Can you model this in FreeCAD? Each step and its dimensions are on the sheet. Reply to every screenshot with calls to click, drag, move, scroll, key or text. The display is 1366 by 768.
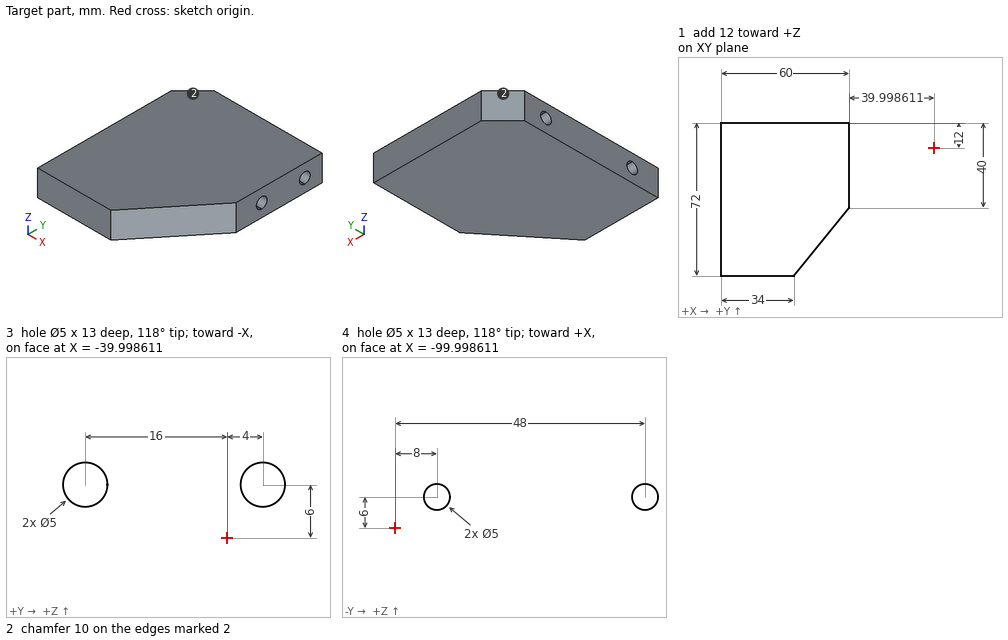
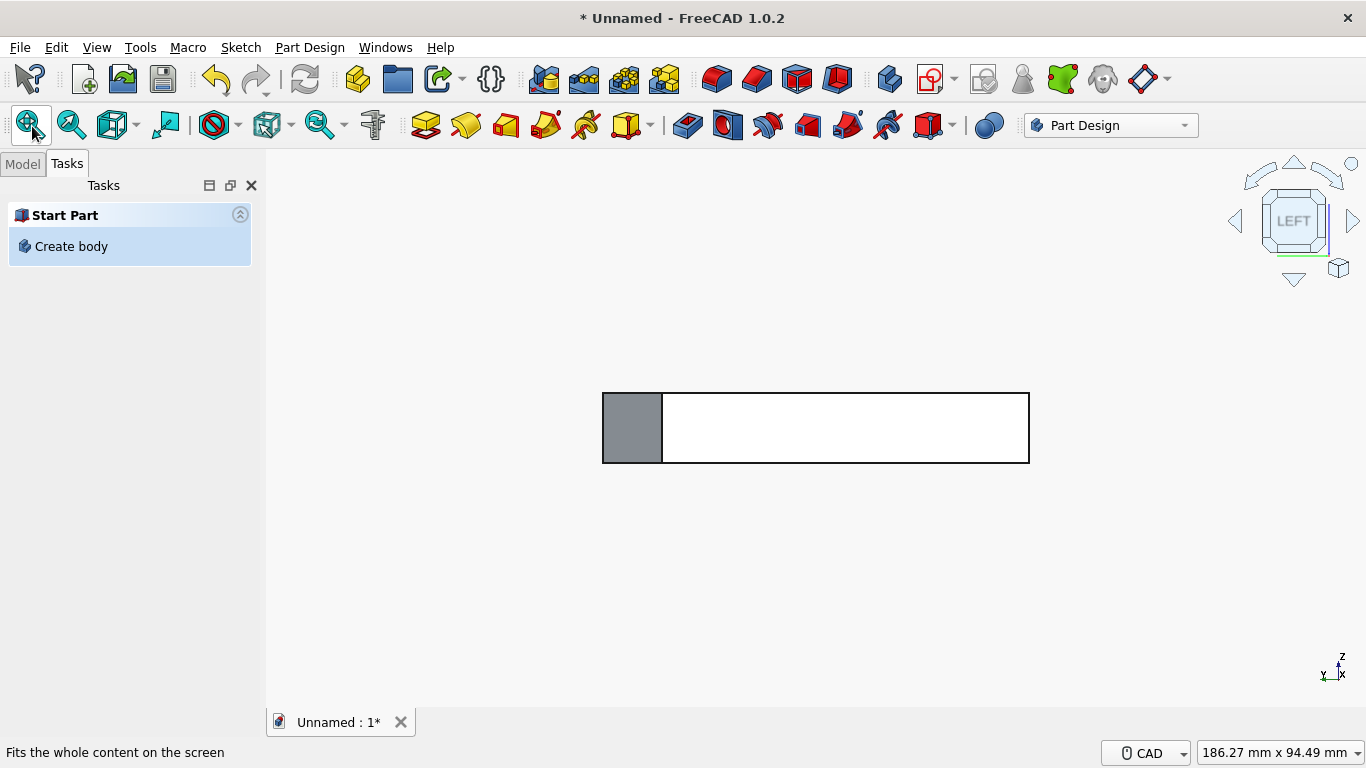
click(741, 427)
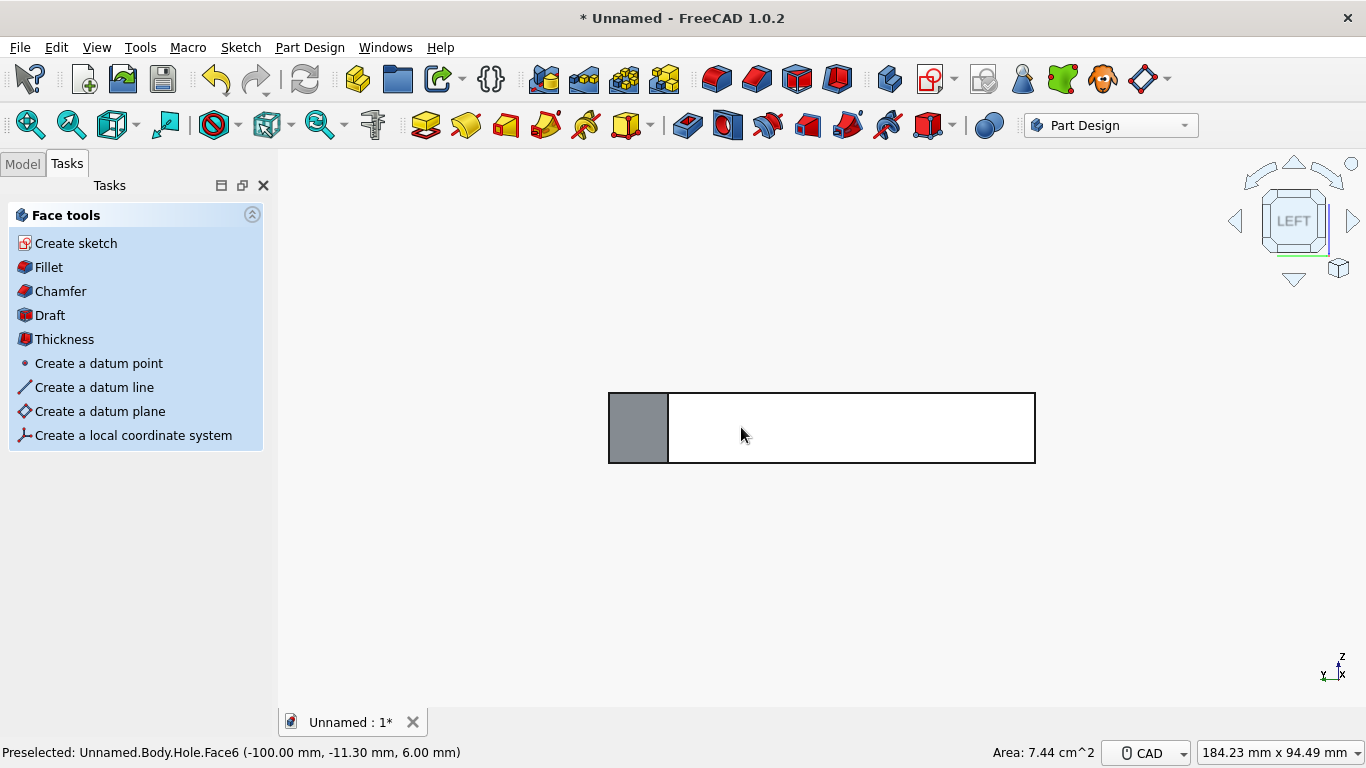
click(930, 80)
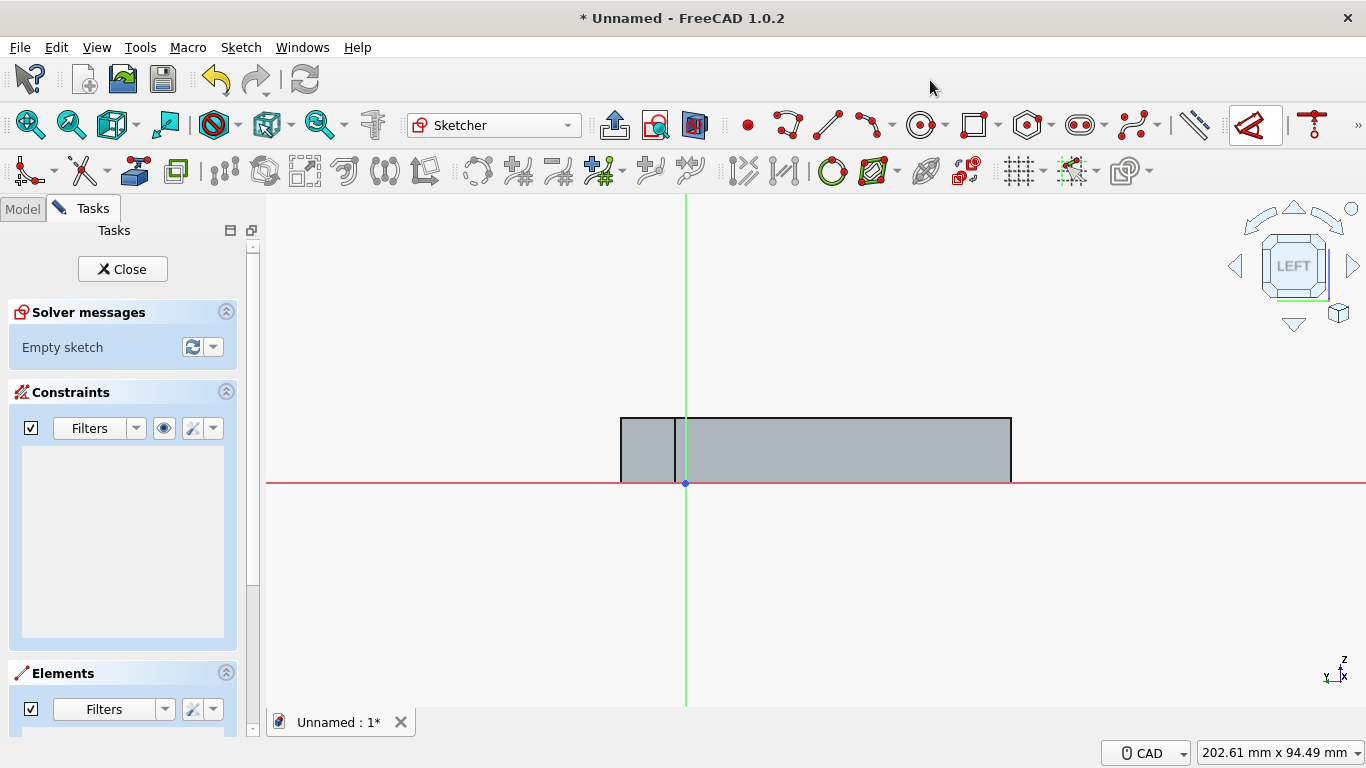
scroll(884, 468, up, 4)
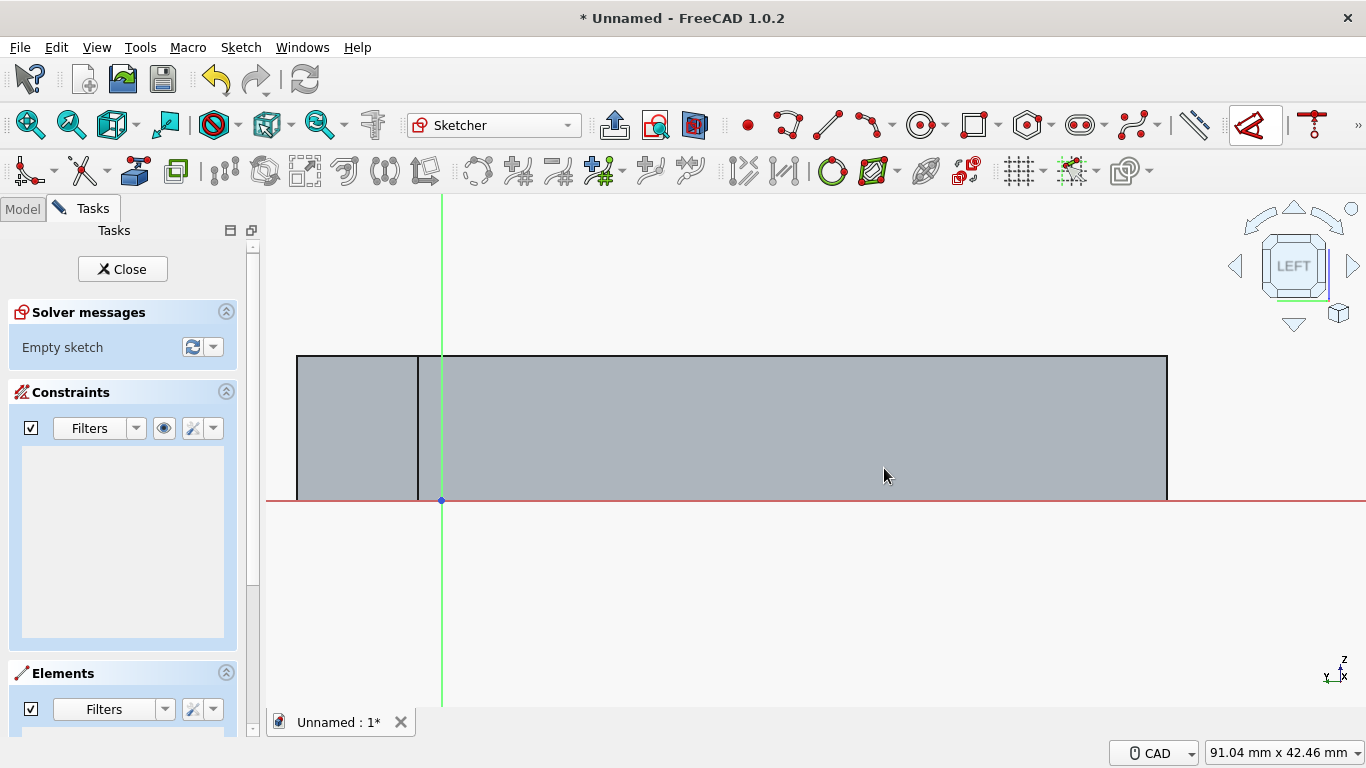
key(g)
key(c)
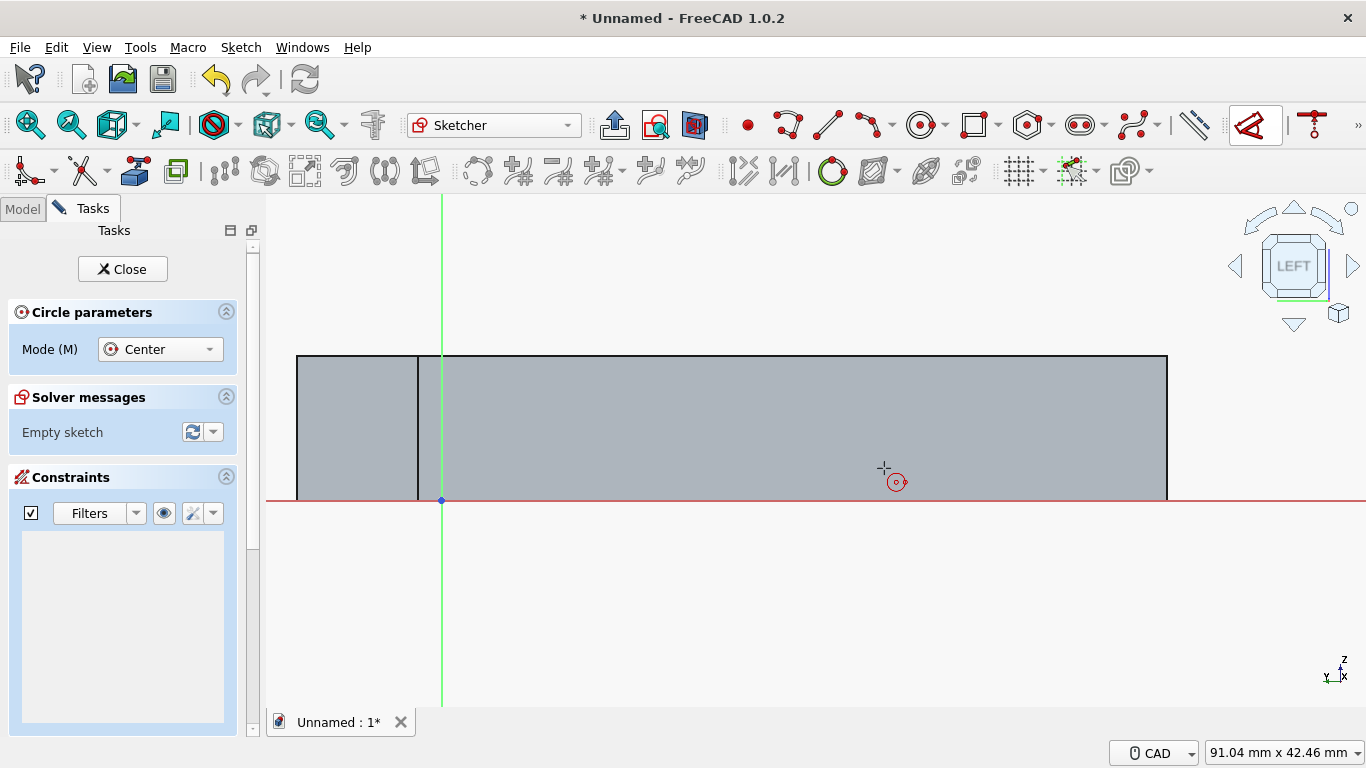
click(539, 428)
move(560, 407)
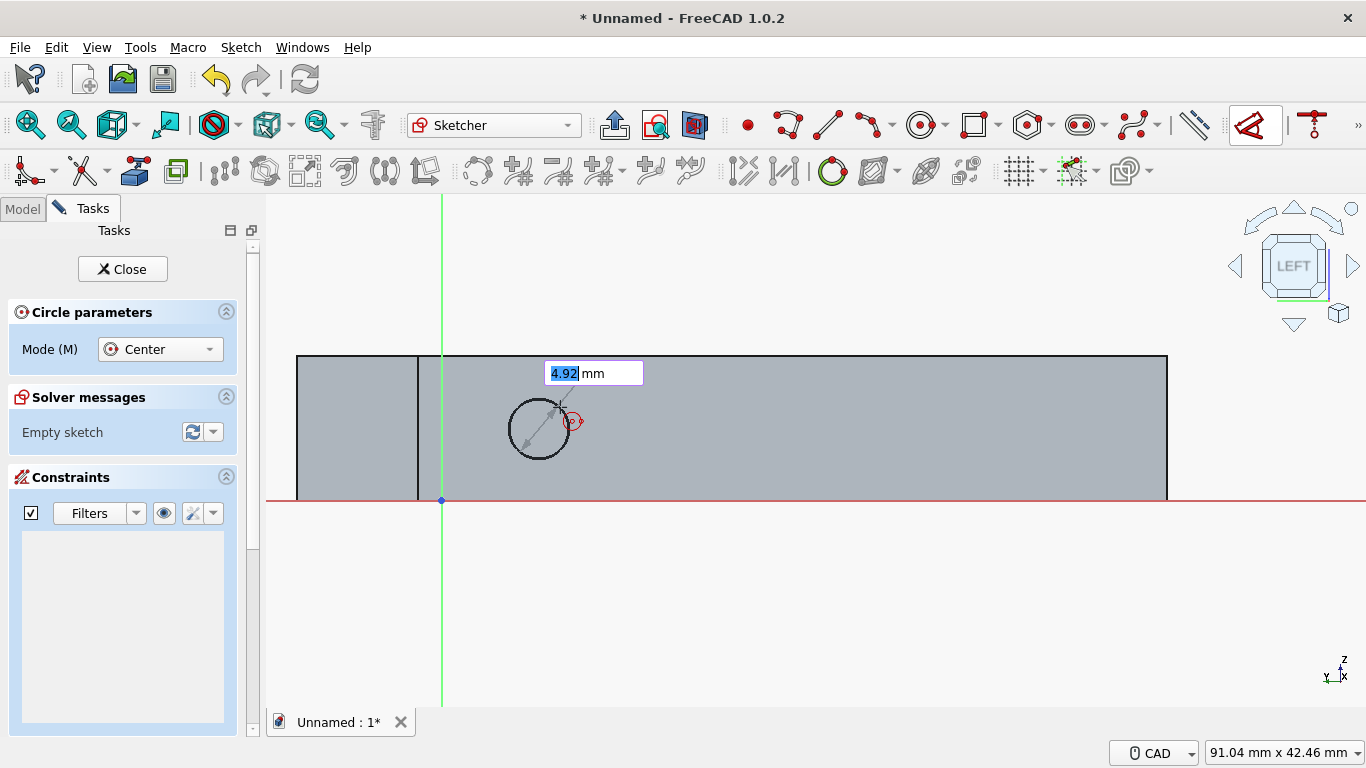
text(5)
key(Return)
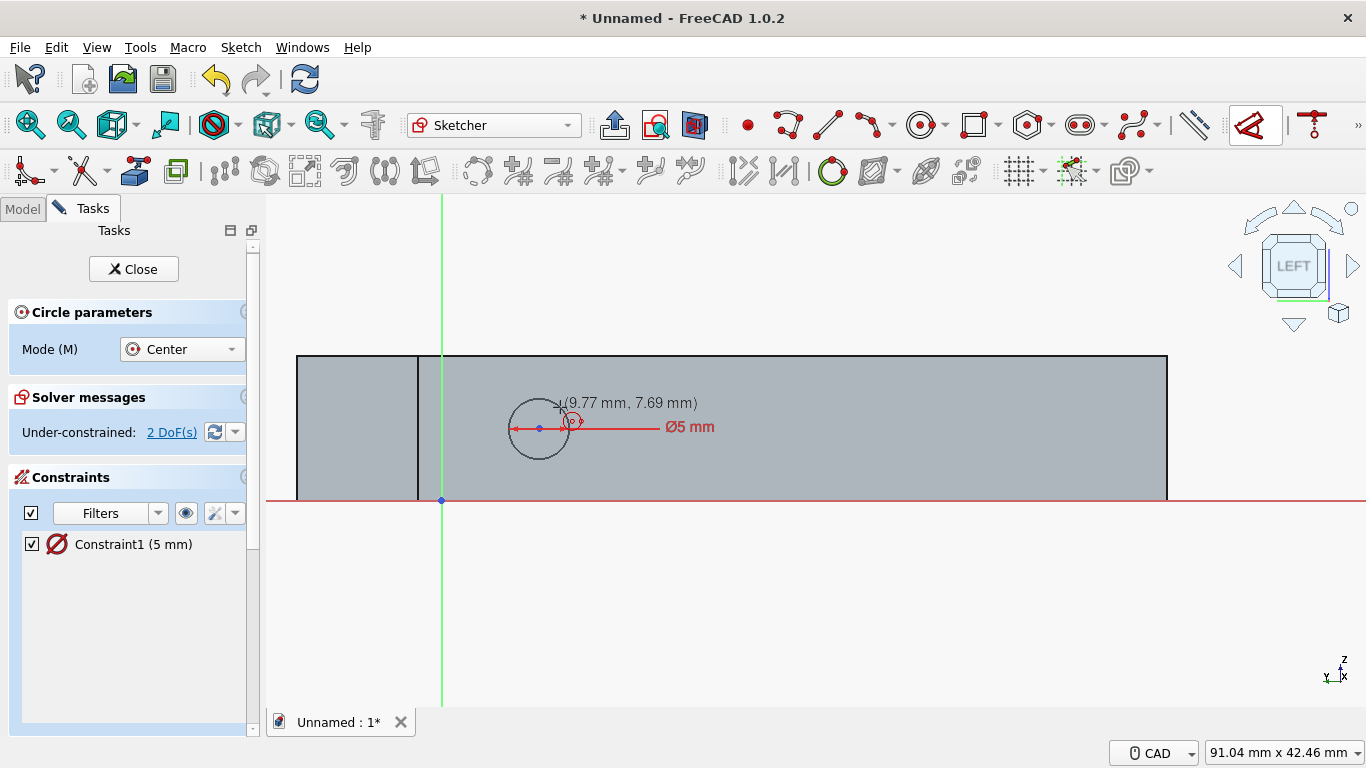
click(1022, 428)
move(1043, 407)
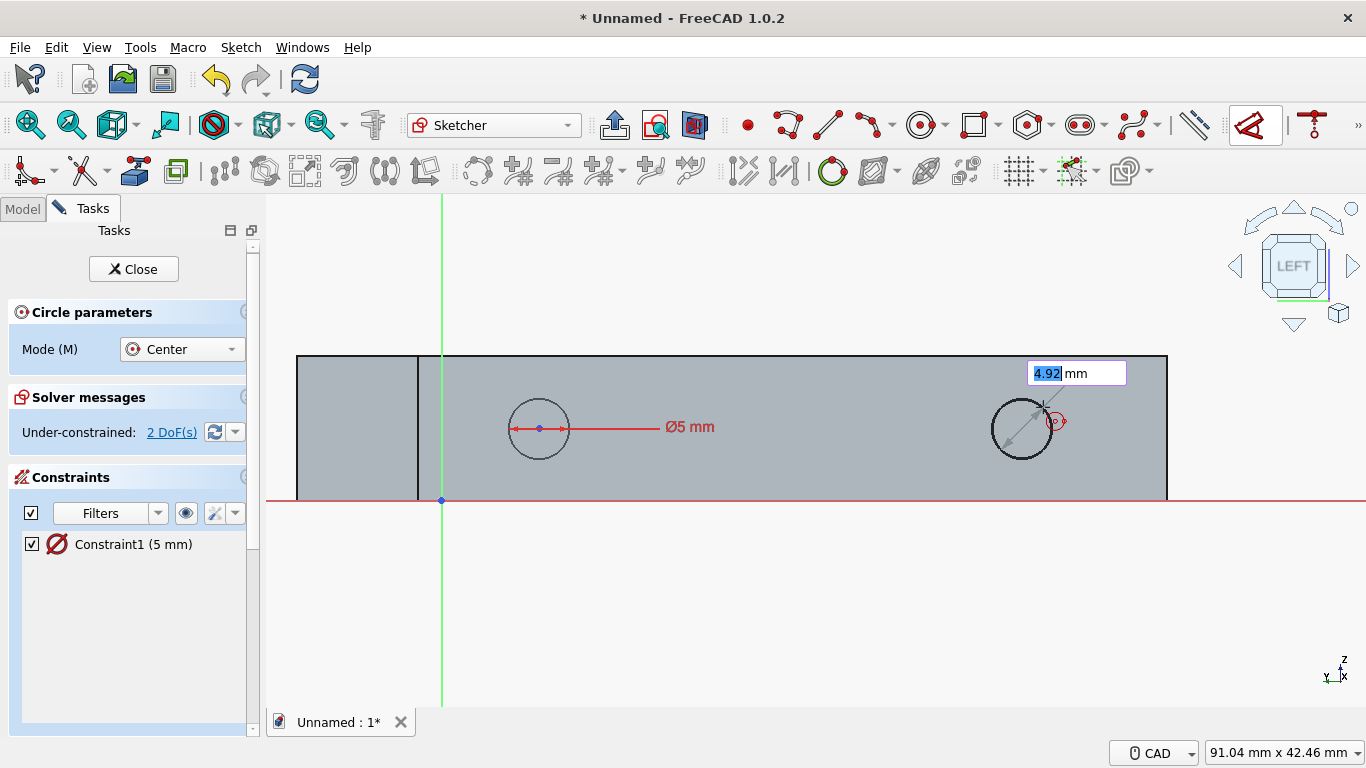
text(5)
key(Return)
key(Escape)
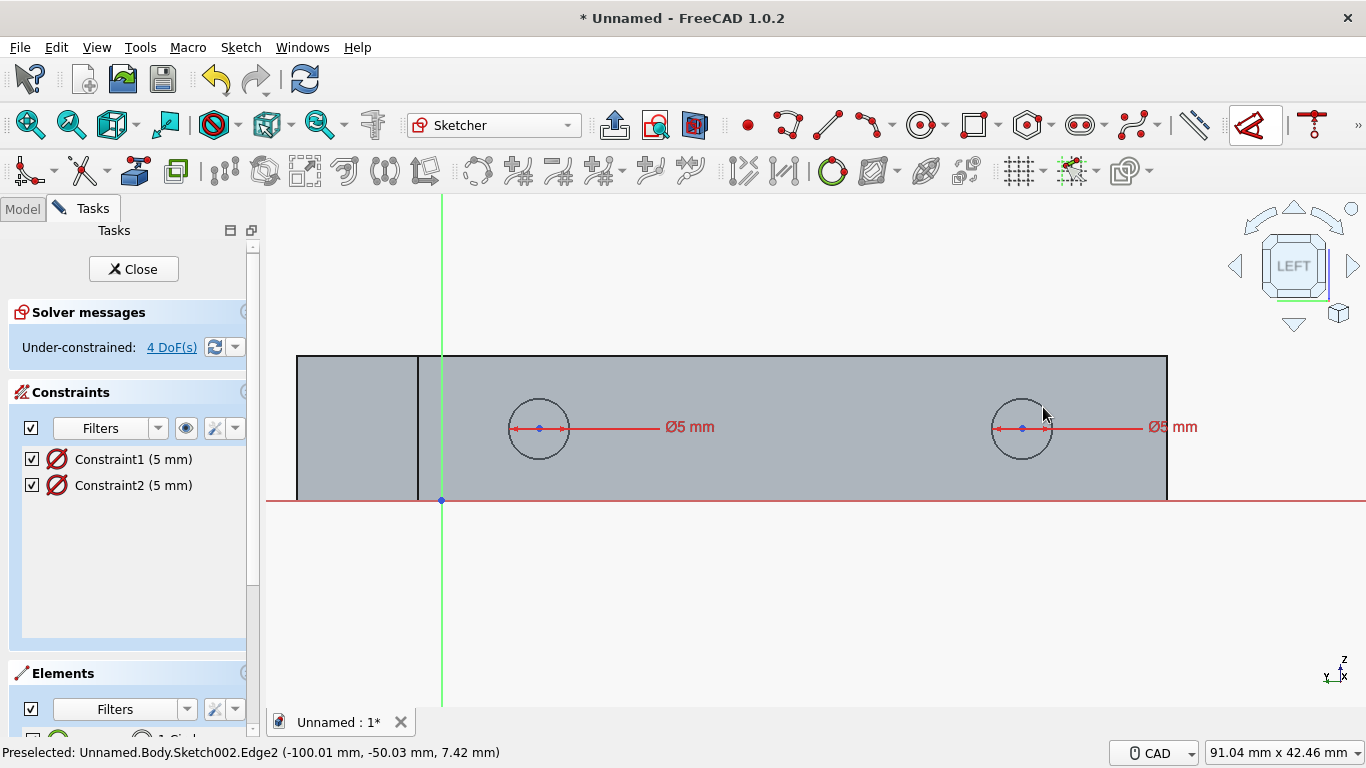
click(539, 429)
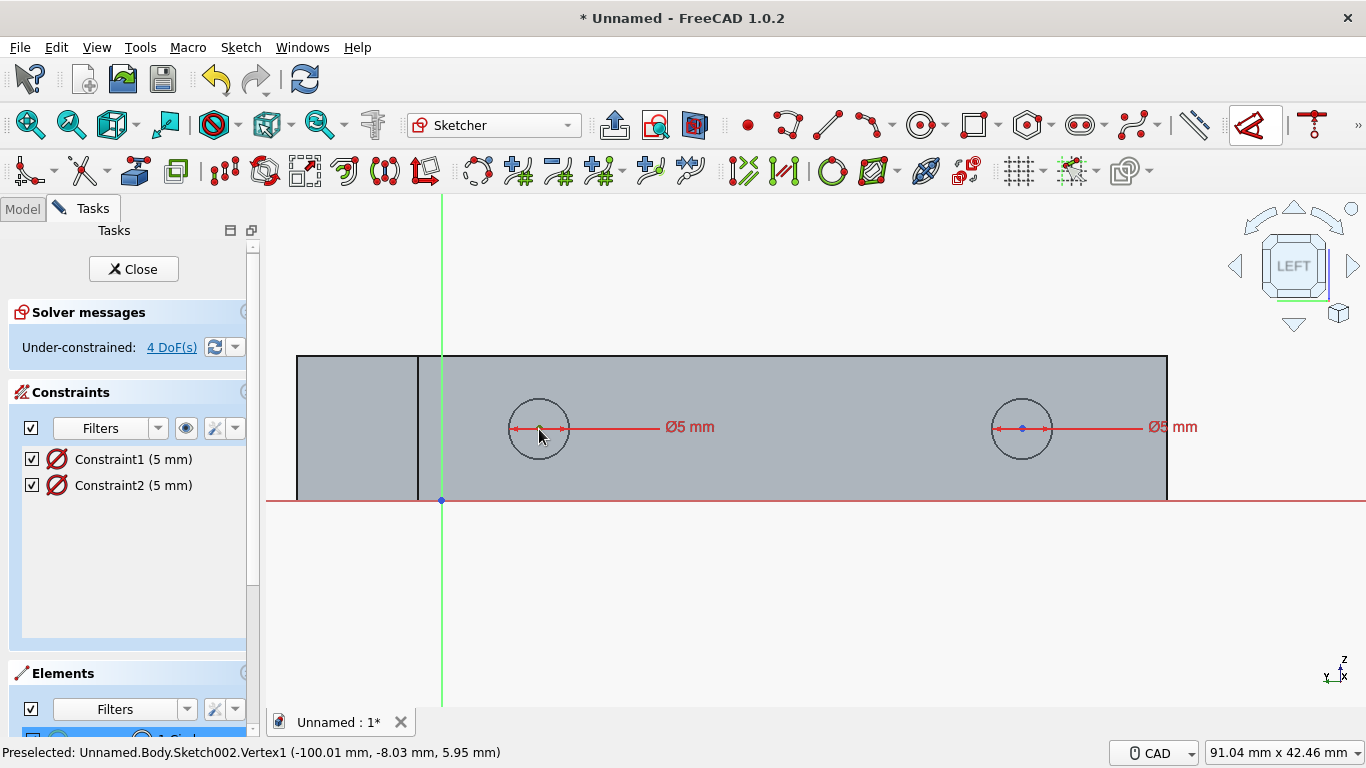
click(1022, 429)